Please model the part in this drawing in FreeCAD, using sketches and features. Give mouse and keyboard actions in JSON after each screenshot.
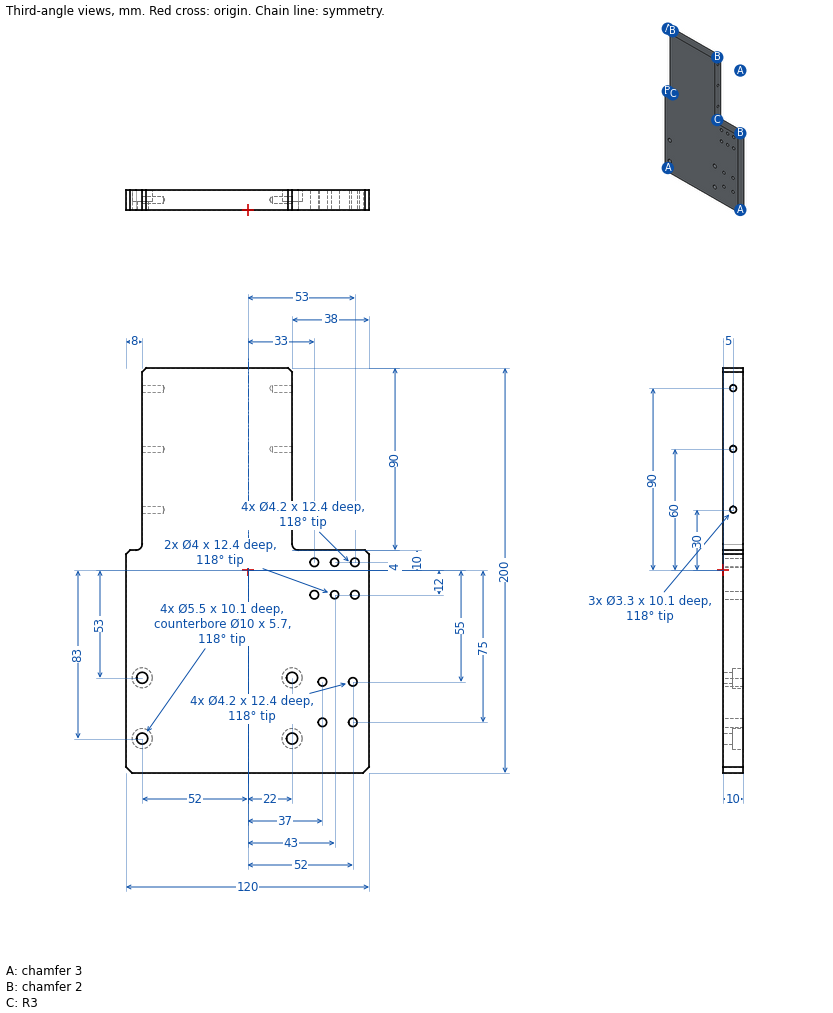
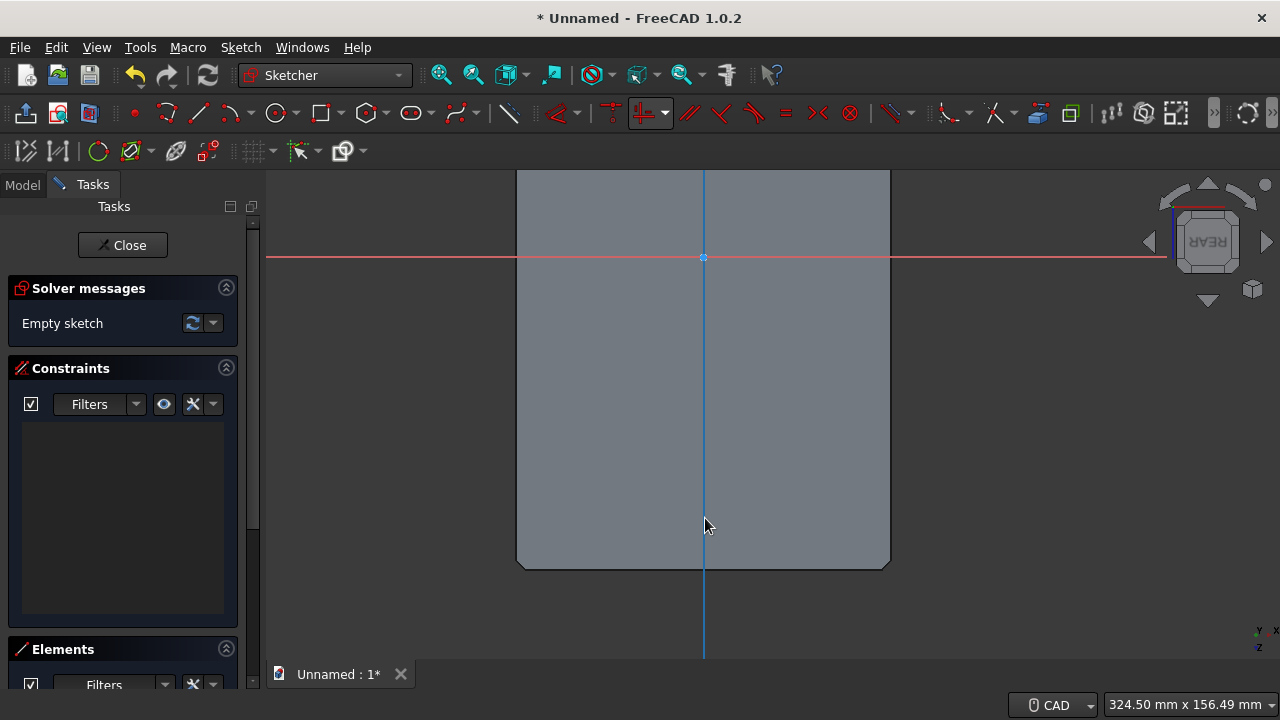
{"action": "left_click", "coordinate": [322, 114]}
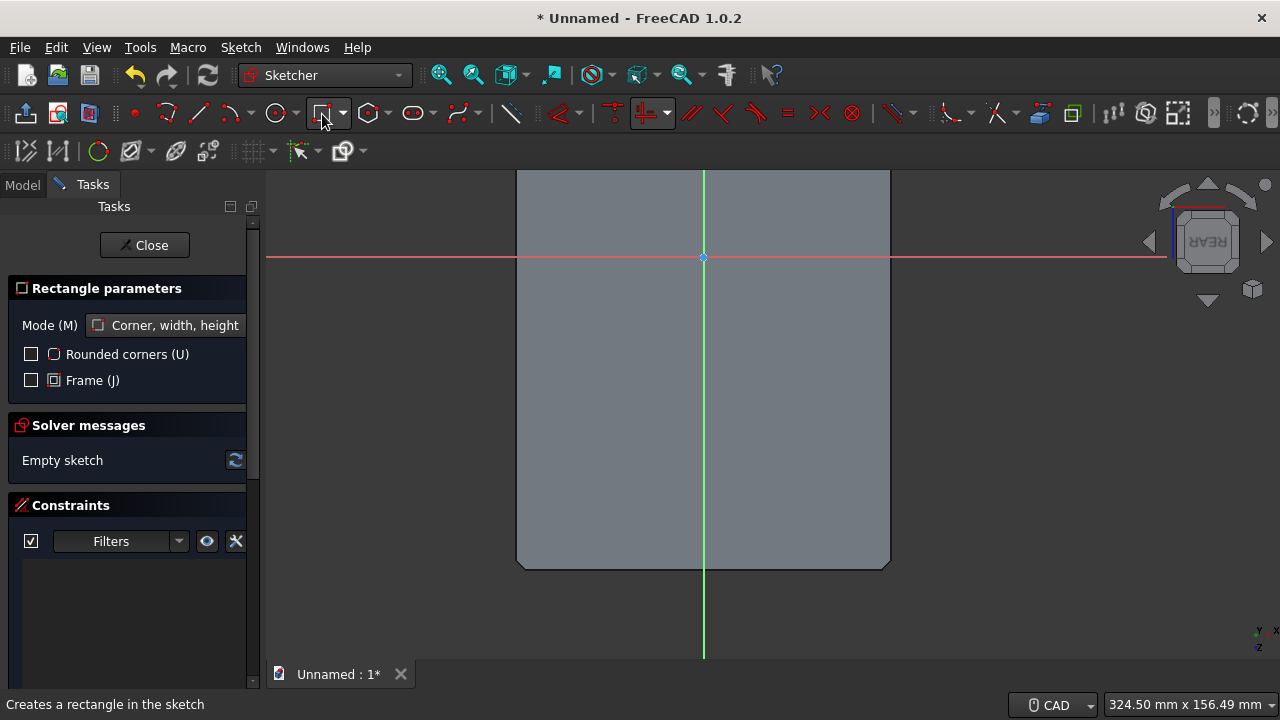
{"action": "left_click", "coordinate": [772, 289]}
{"action": "left_click", "coordinate": [891, 570]}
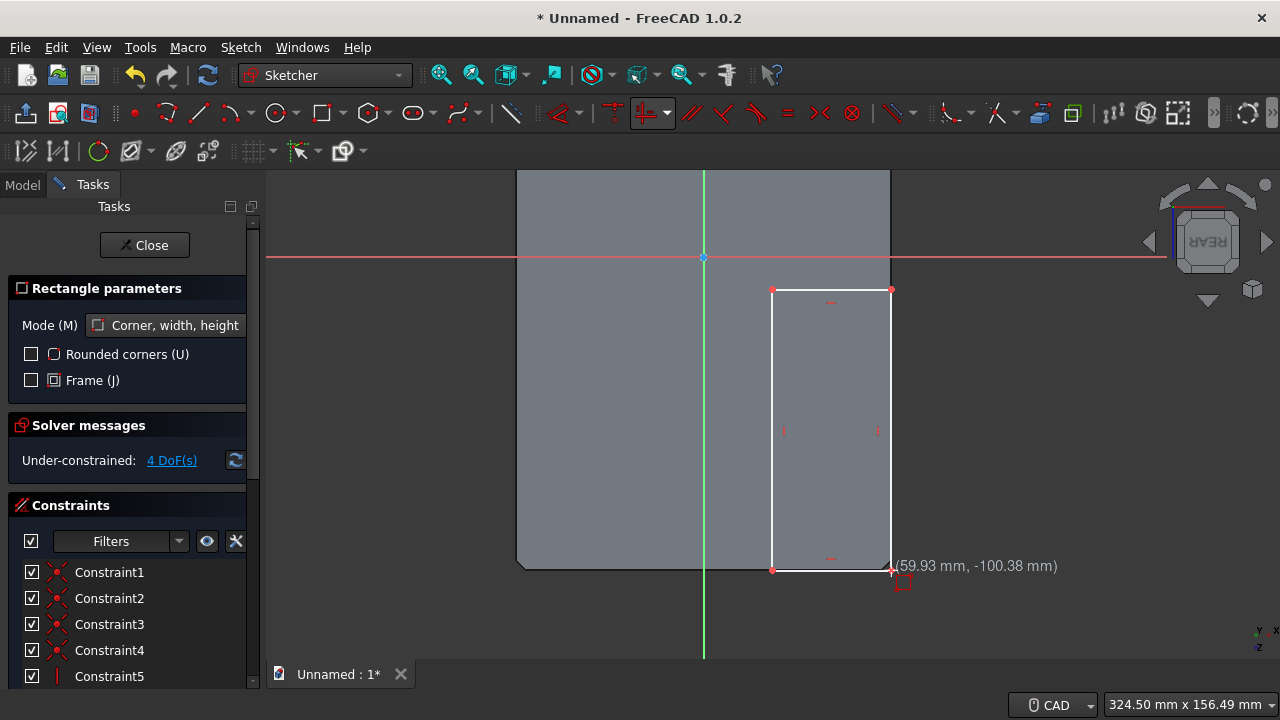
{"action": "left_click", "coordinate": [516, 289]}
{"action": "left_click", "coordinate": [541, 570]}
{"action": "key", "text": "Escape"}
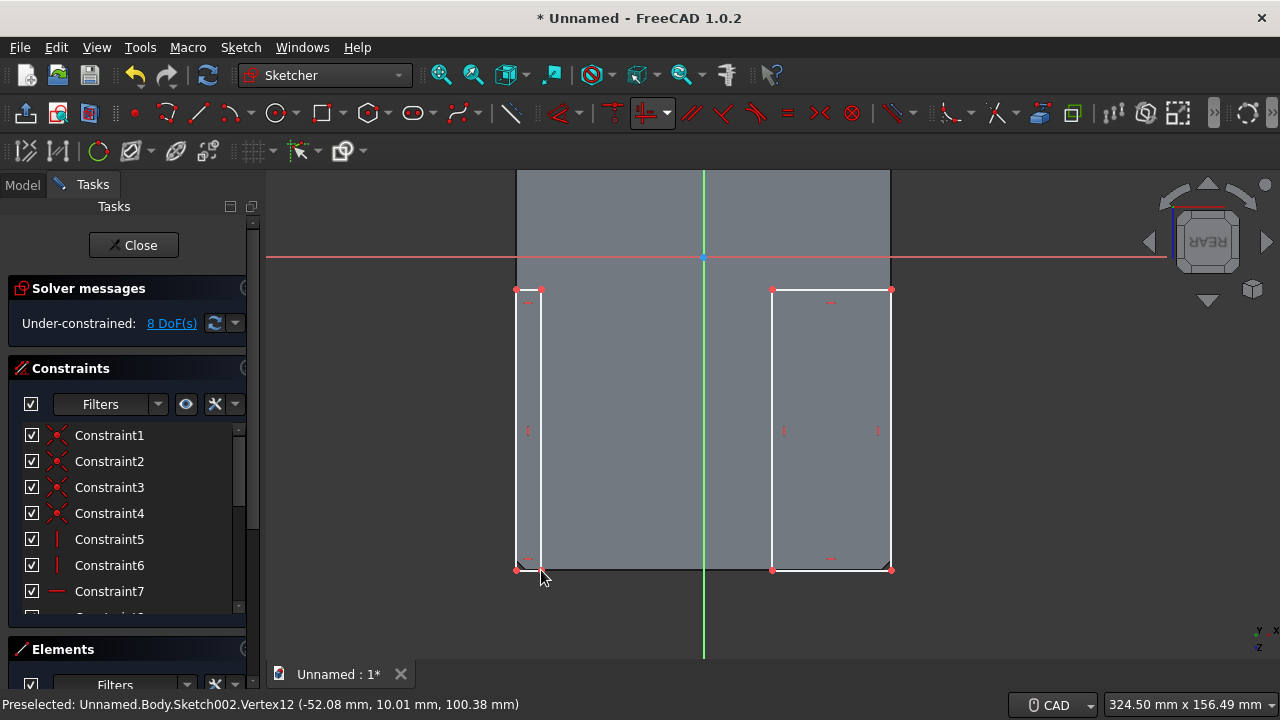
{"action": "left_click", "coordinate": [891, 290]}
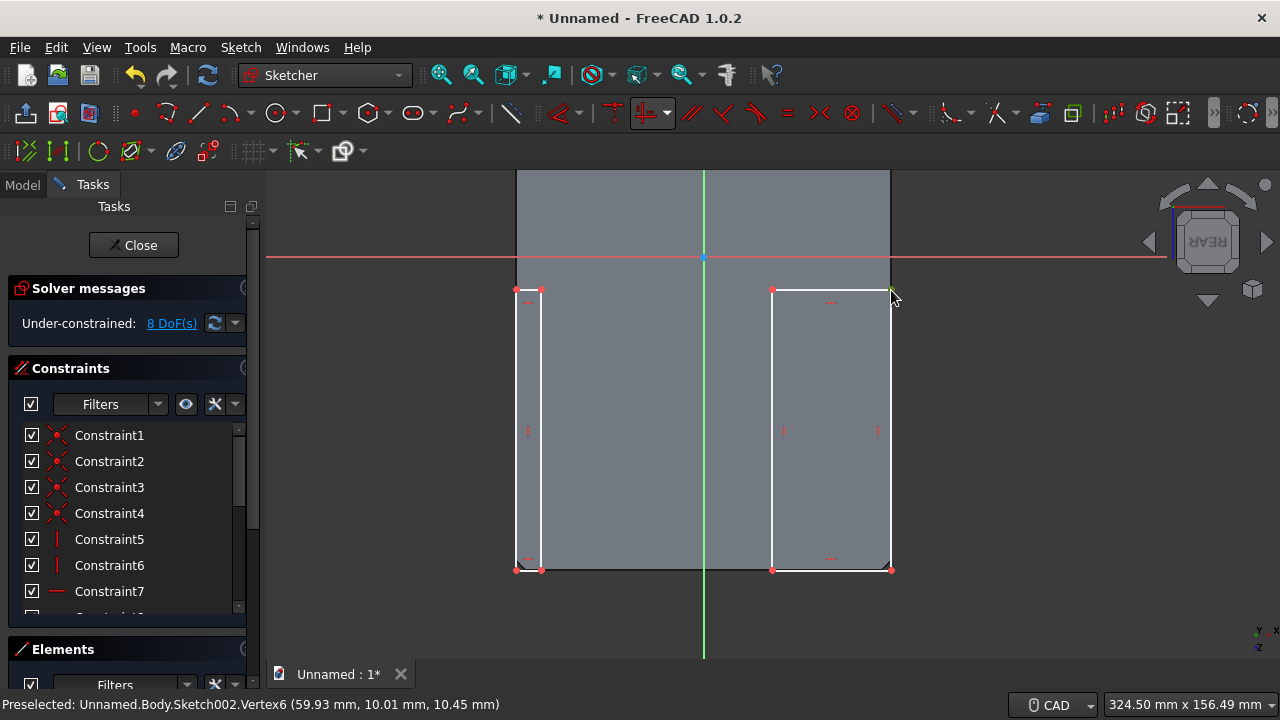
{"action": "left_click", "coordinate": [516, 290]}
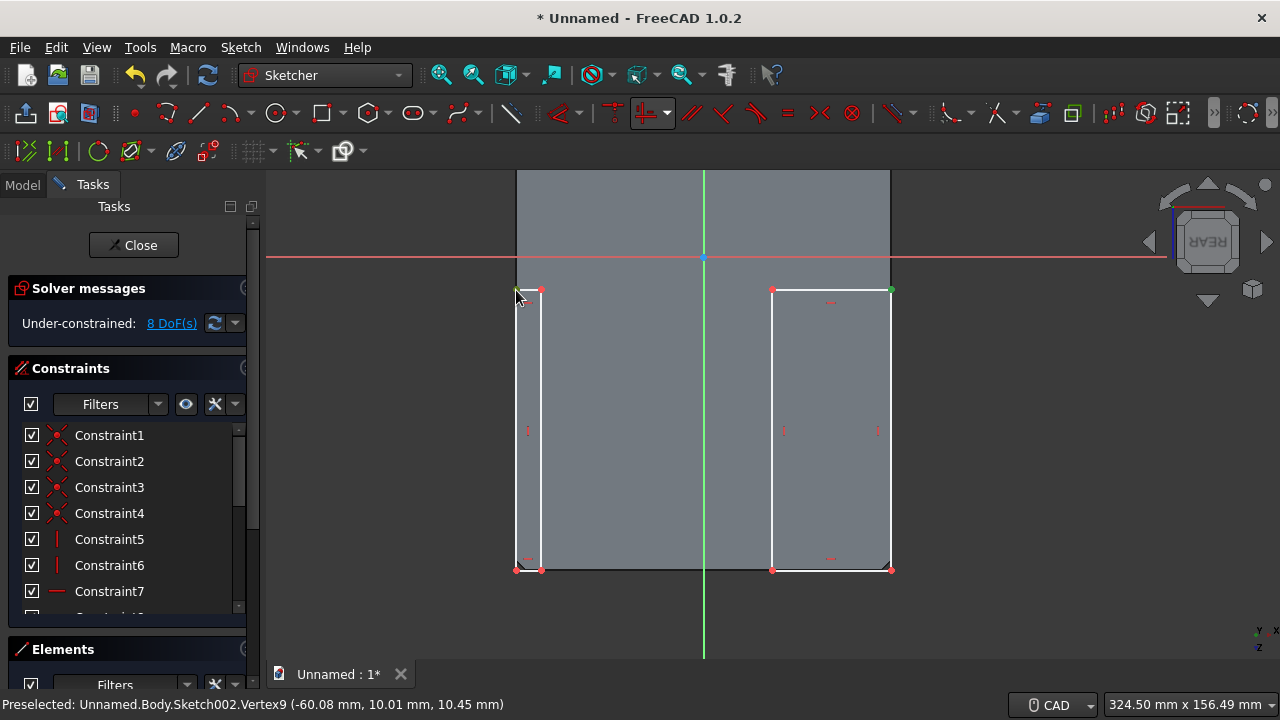
{"action": "left_click", "coordinate": [704, 600]}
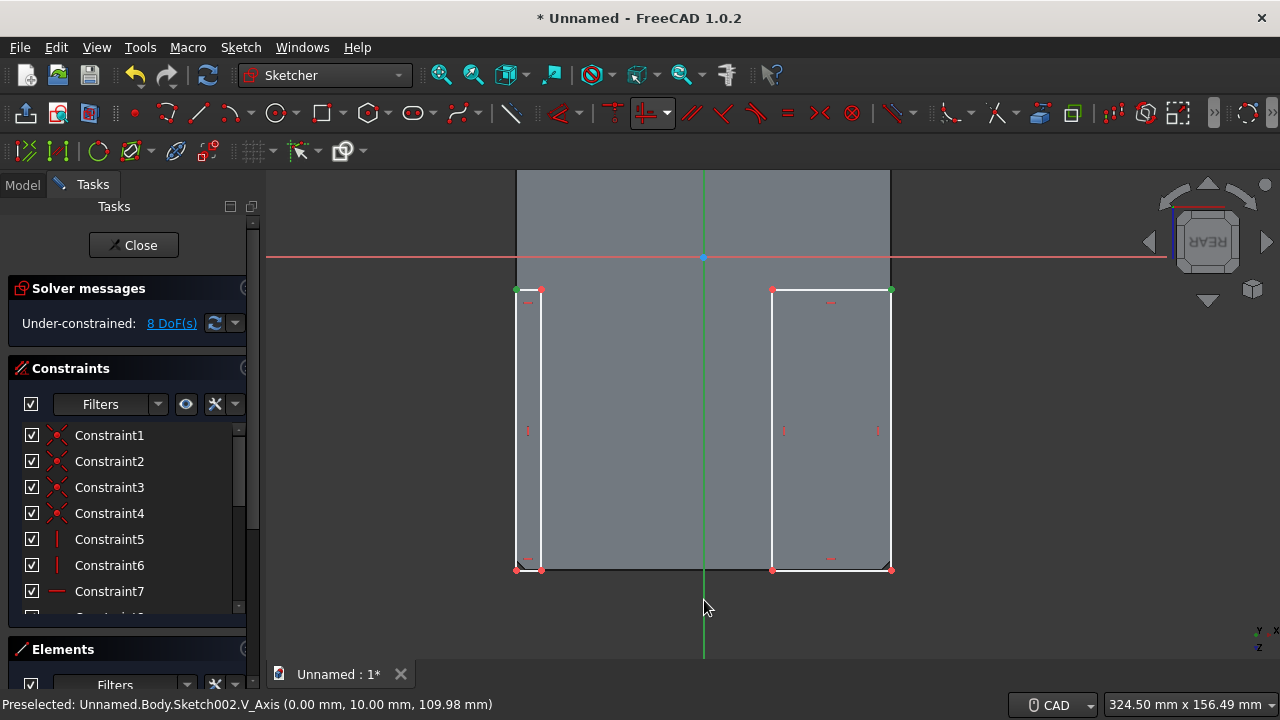
{"action": "left_click", "coordinate": [820, 114]}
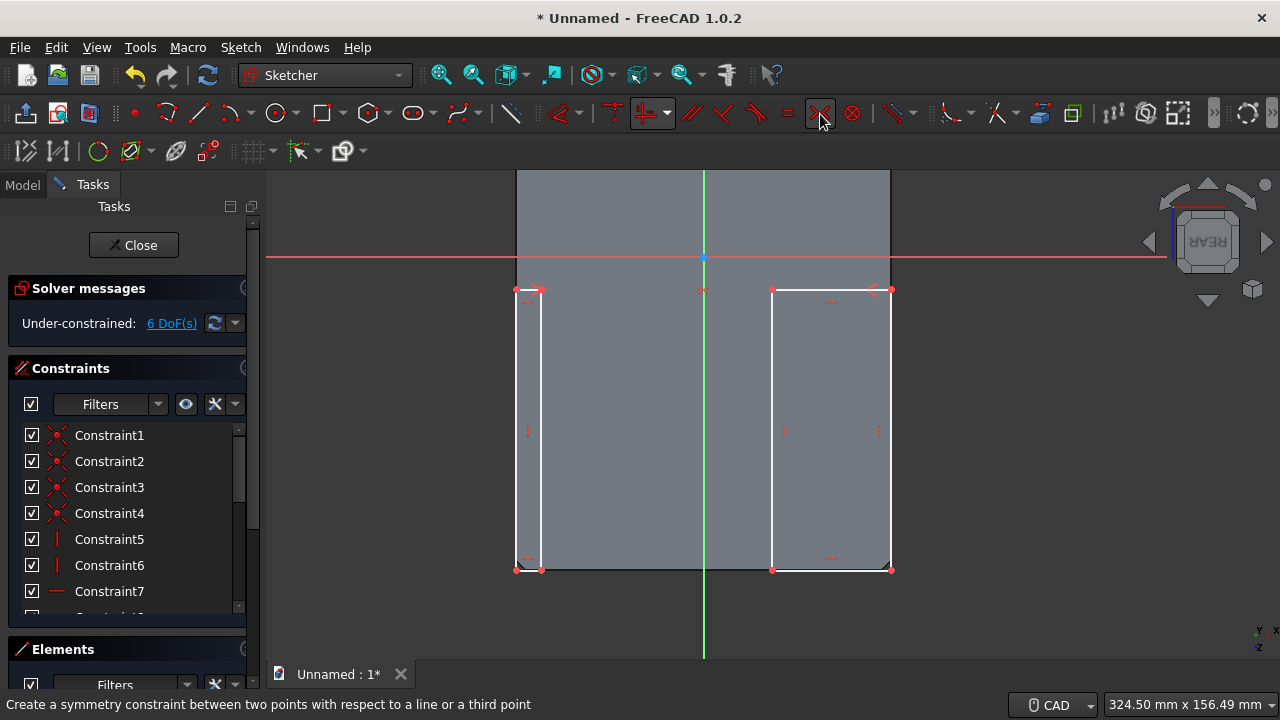
{"action": "left_click", "coordinate": [558, 114]}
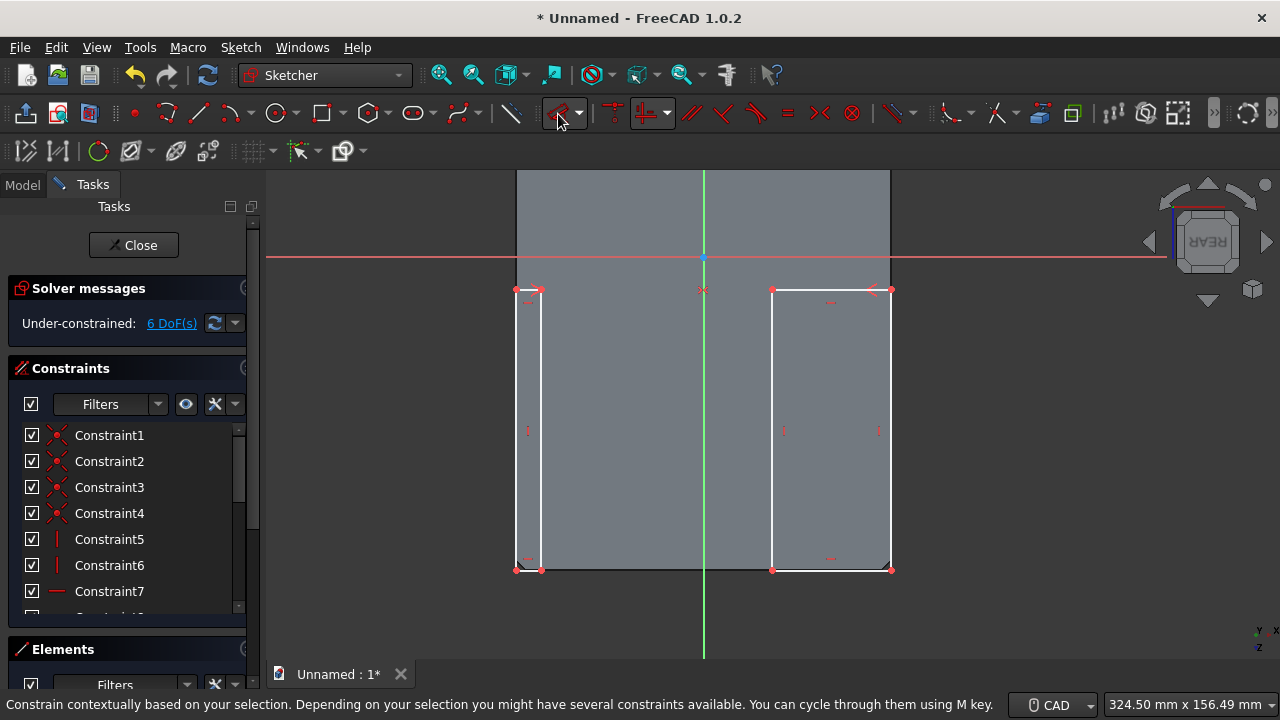
{"action": "scroll", "coordinate": [526, 571], "scroll_direction": "up", "scroll_amount": 3}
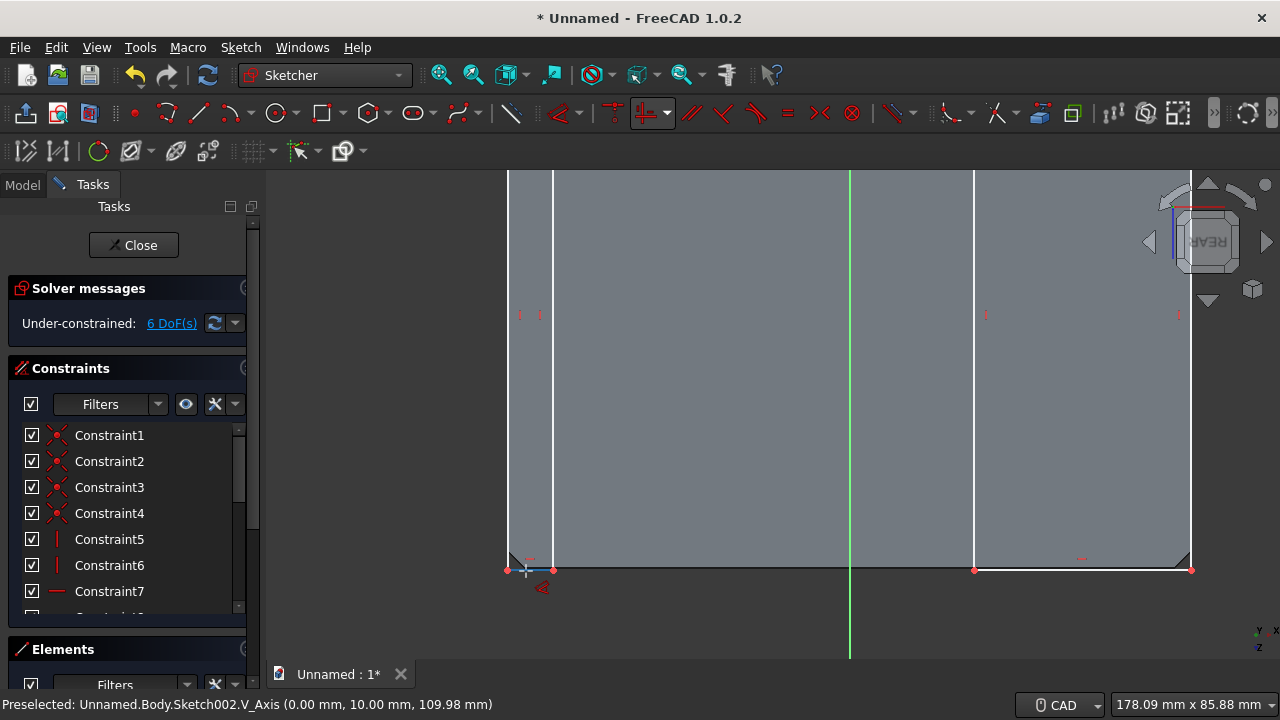
{"action": "left_click", "coordinate": [526, 570]}
{"action": "left_click", "coordinate": [531, 604]}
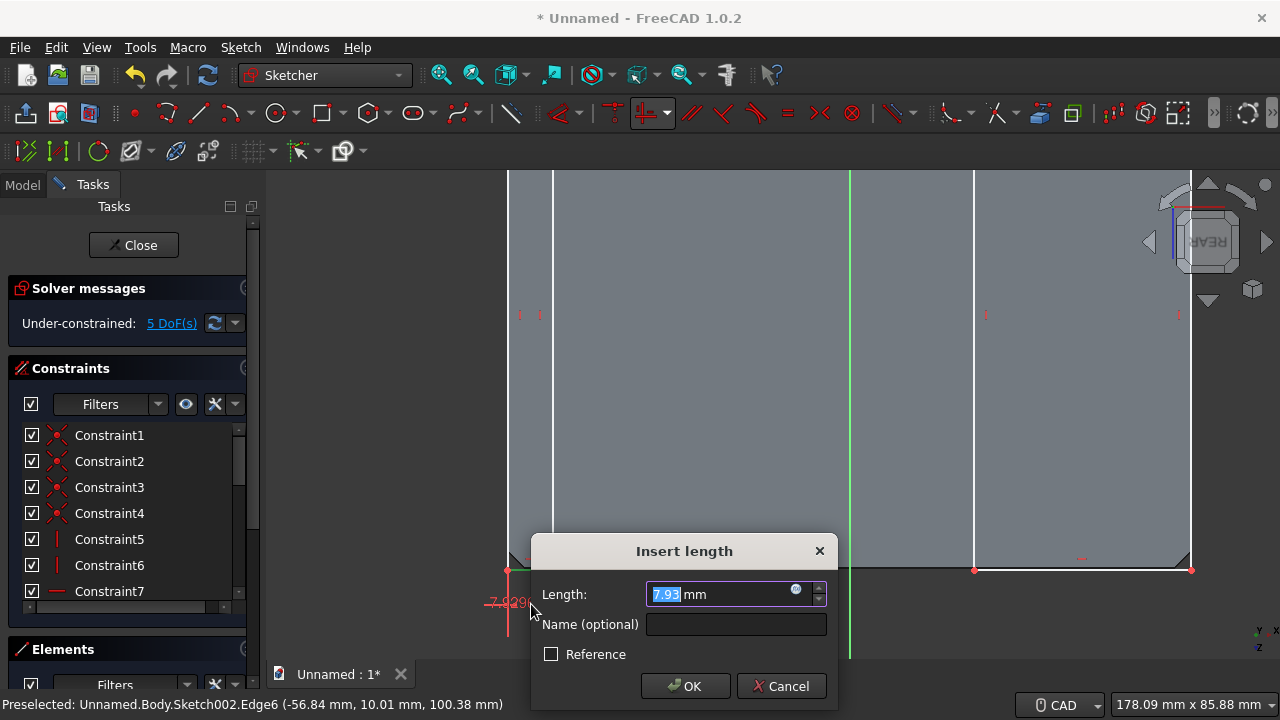
{"action": "type", "text": "8"}
{"action": "key", "text": "Return"}